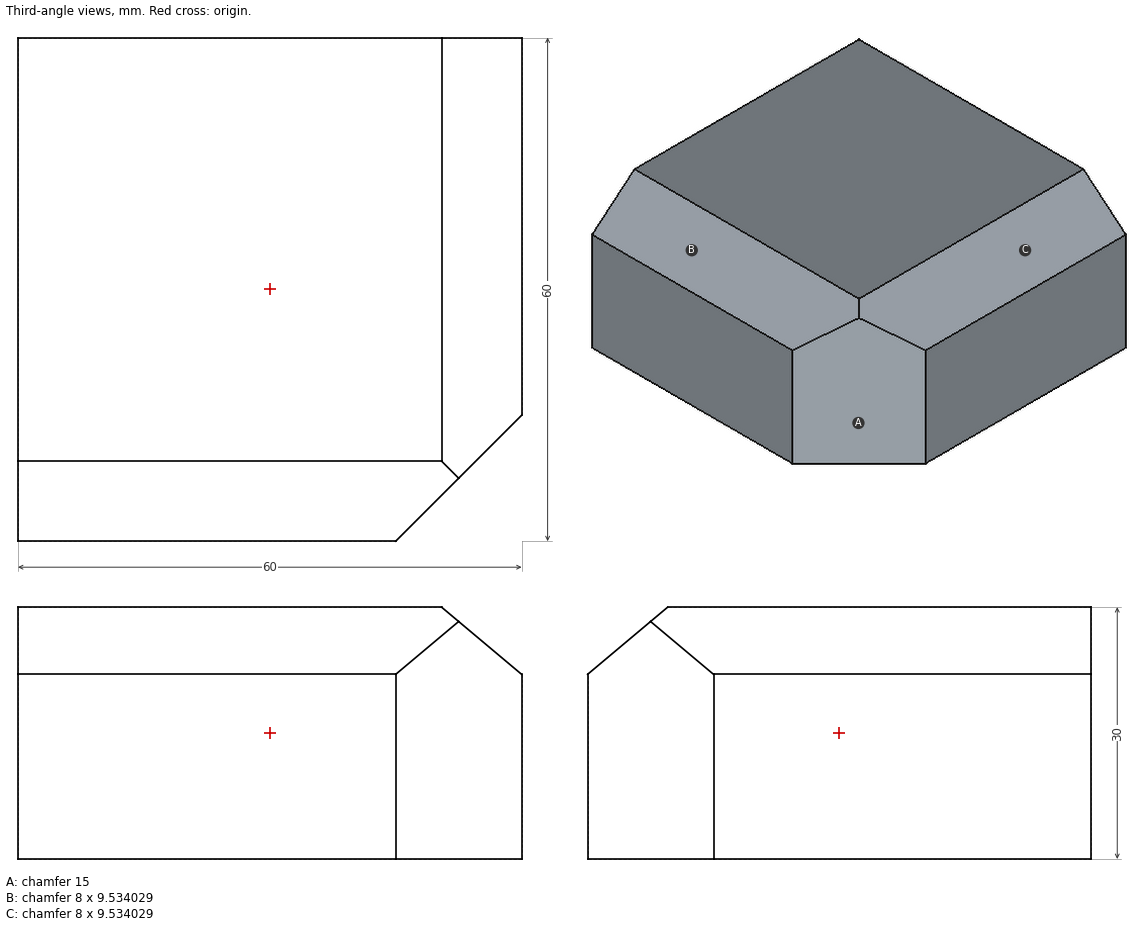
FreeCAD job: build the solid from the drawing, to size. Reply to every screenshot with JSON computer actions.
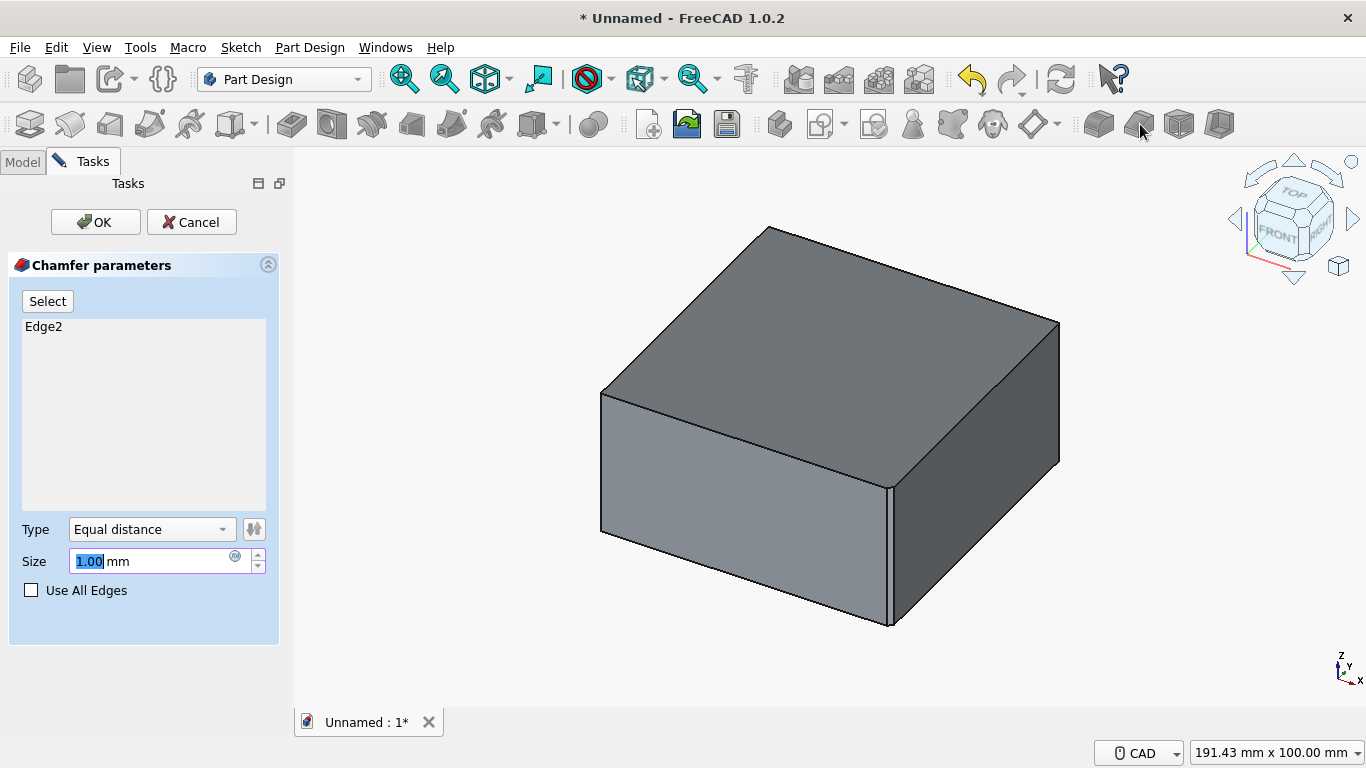
{"action": "type", "text": "15"}
{"action": "key", "text": "Tab"}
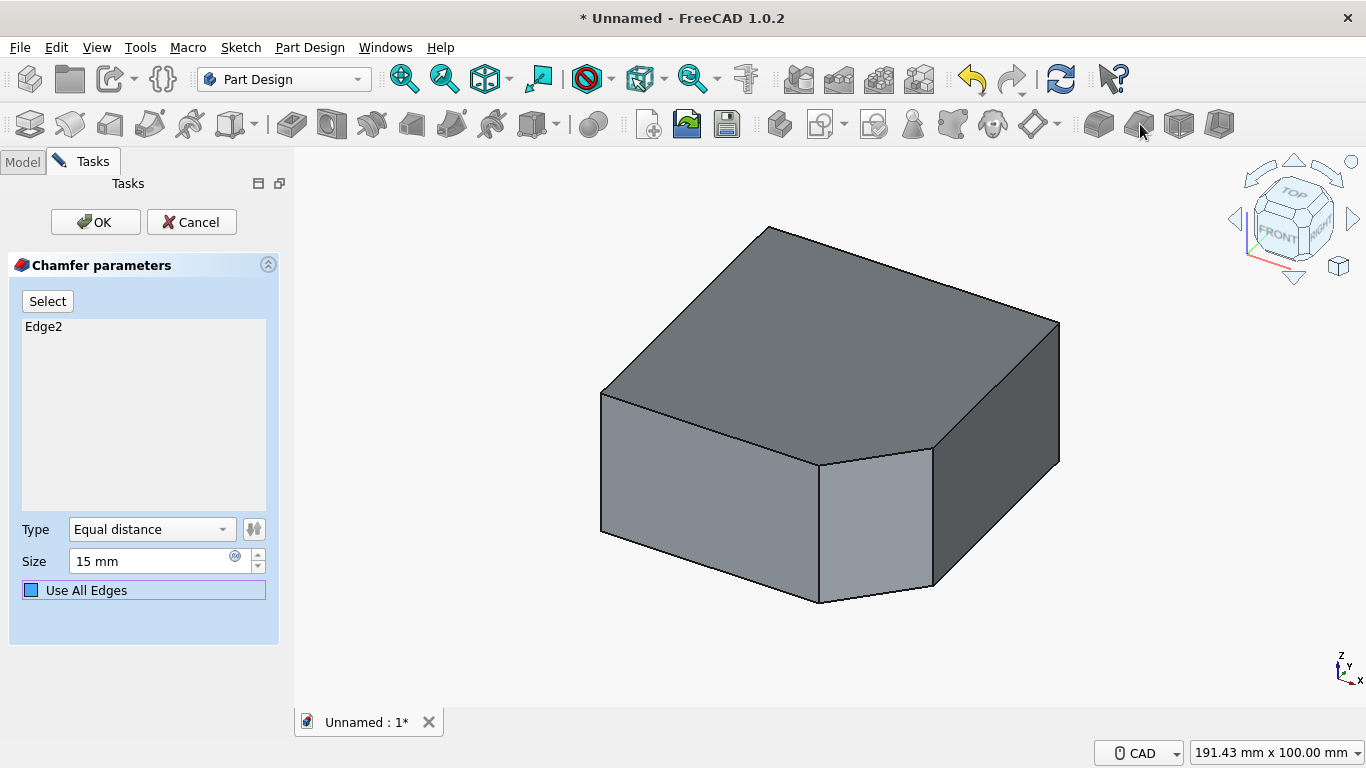
{"action": "left_click", "coordinate": [96, 222]}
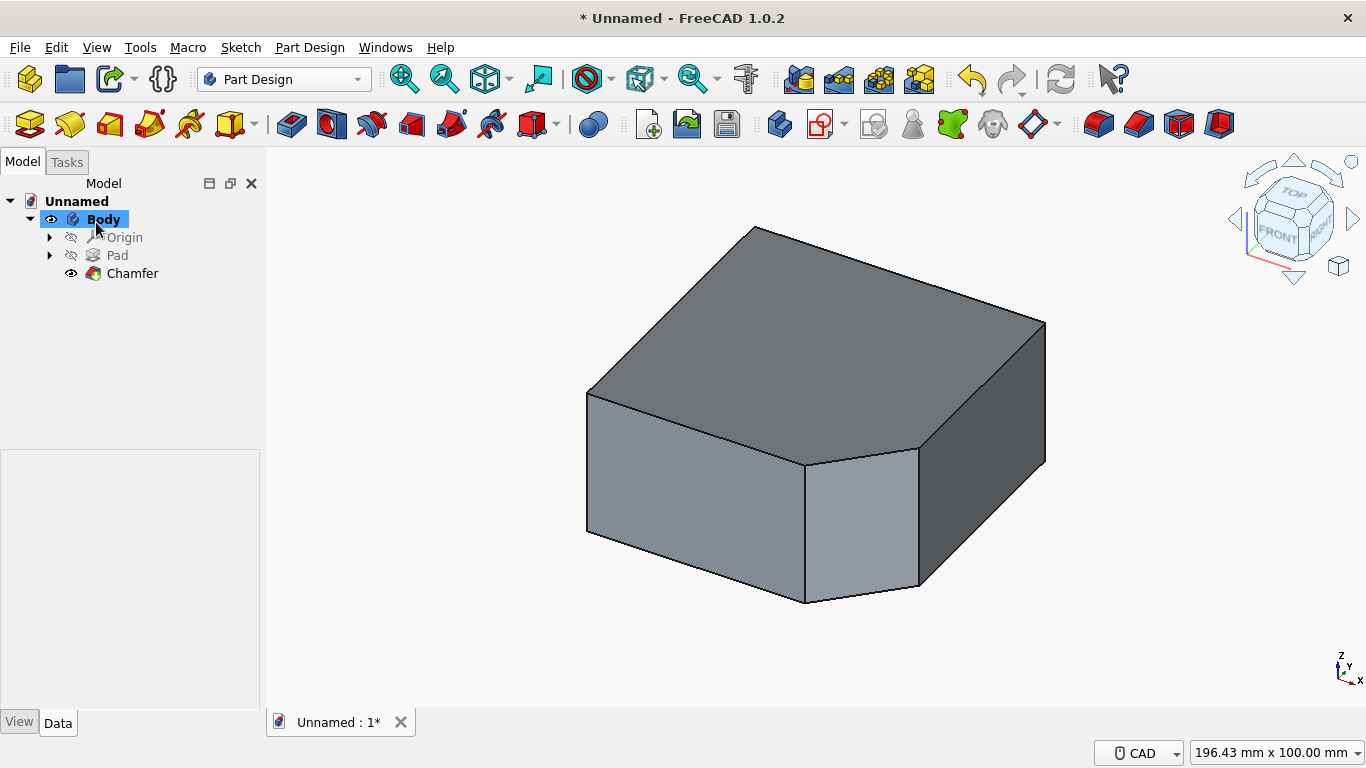
{"action": "left_click", "coordinate": [696, 429]}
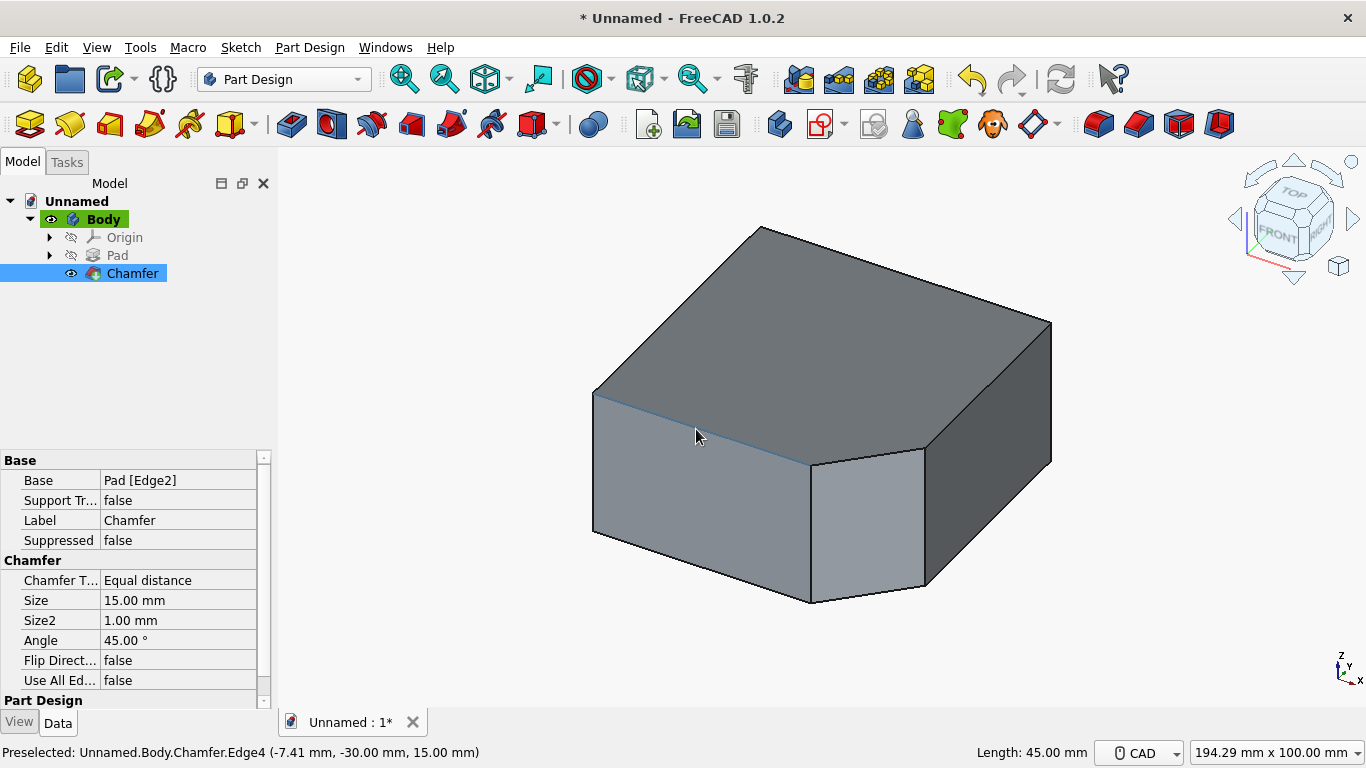
{"action": "left_click", "coordinate": [1140, 124]}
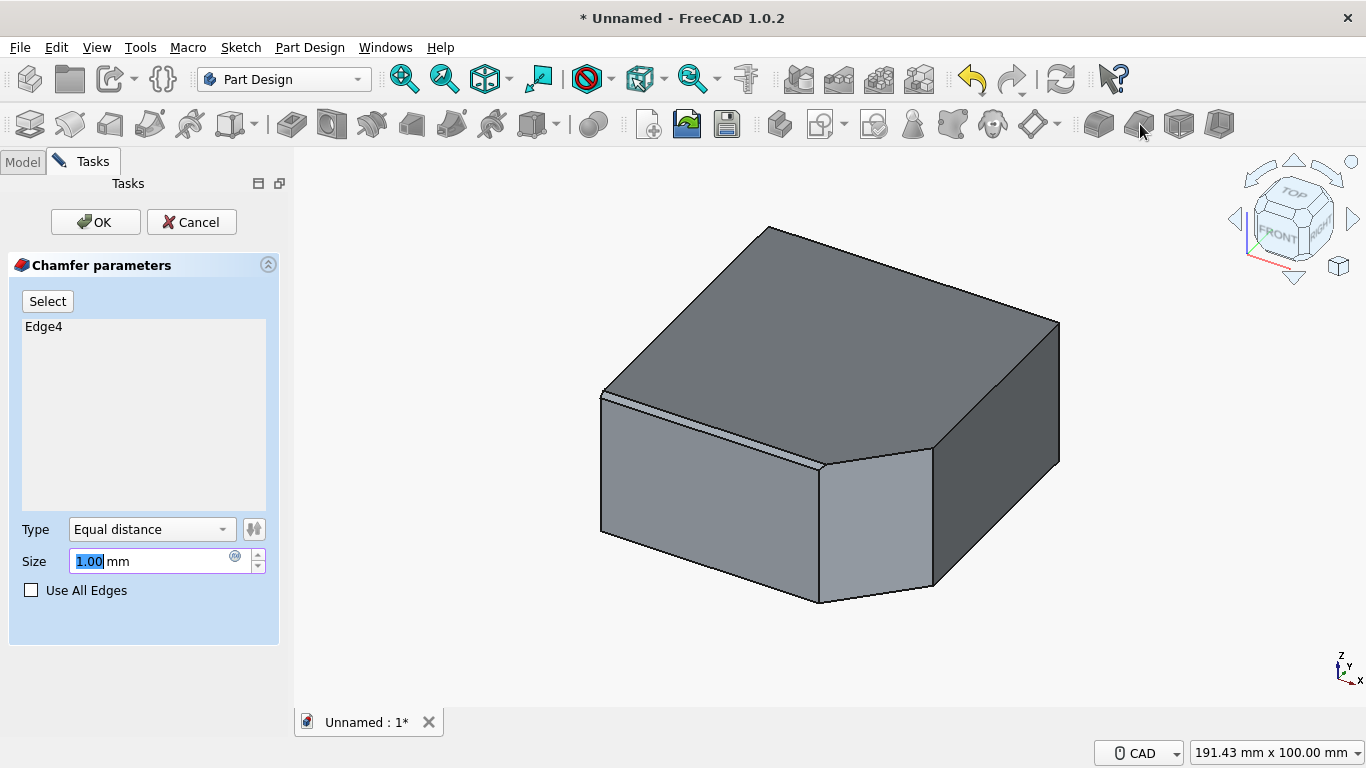
{"action": "type", "text": "8"}
{"action": "key", "text": "Tab"}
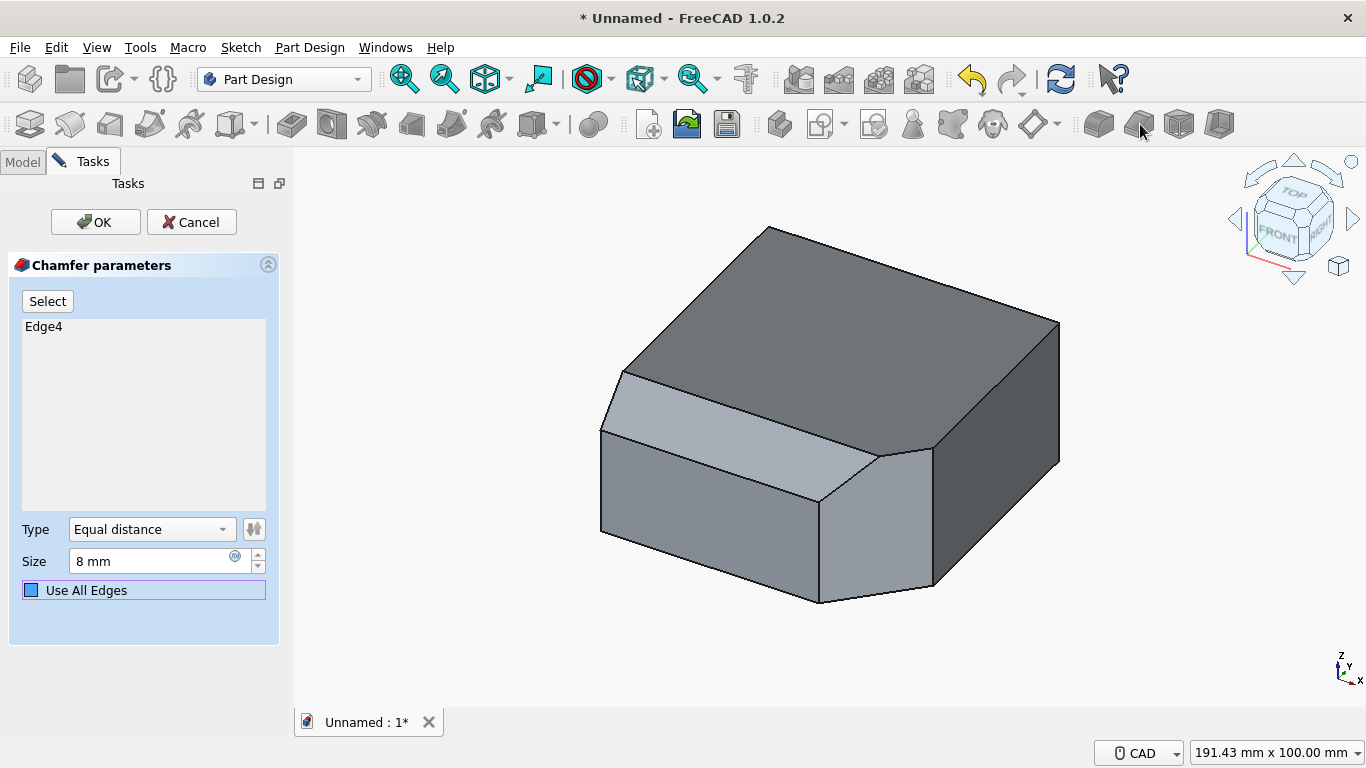
{"action": "left_click", "coordinate": [153, 530]}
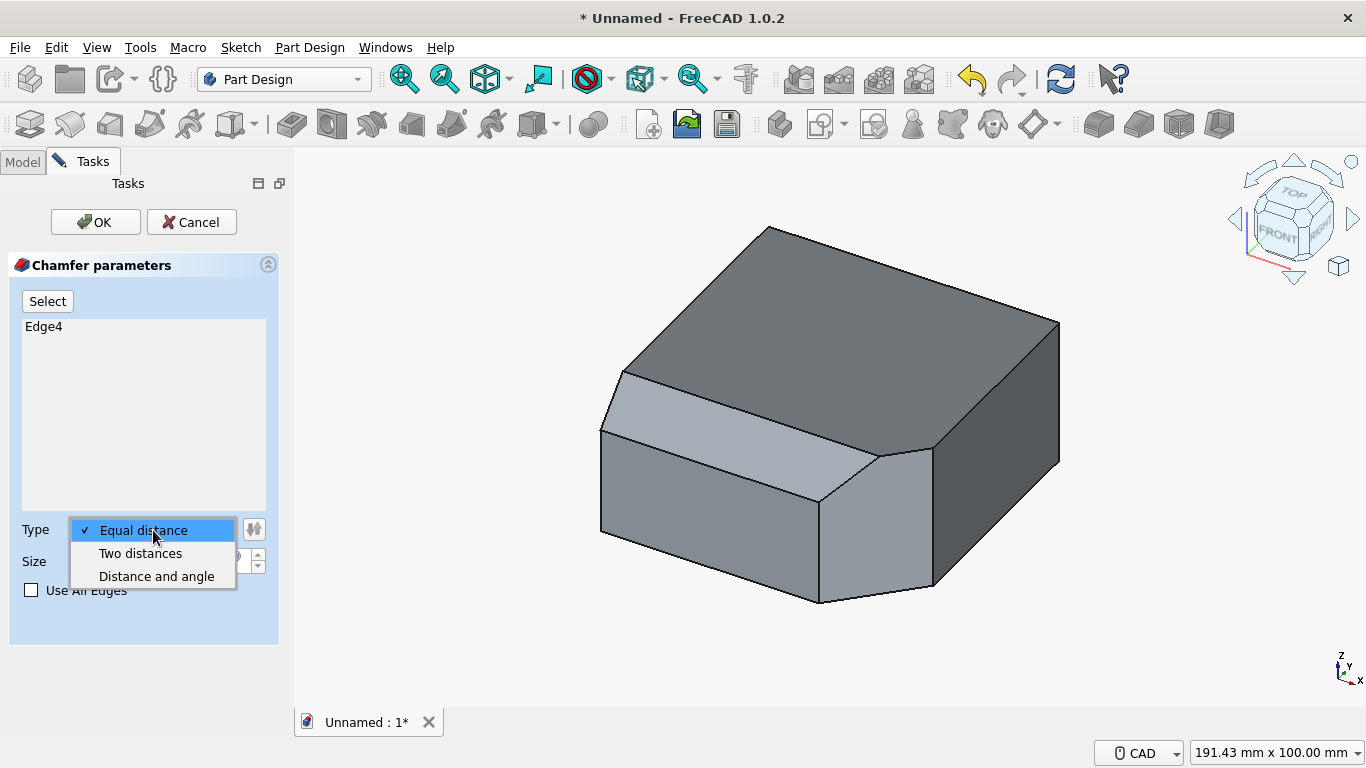
{"action": "left_click", "coordinate": [152, 554]}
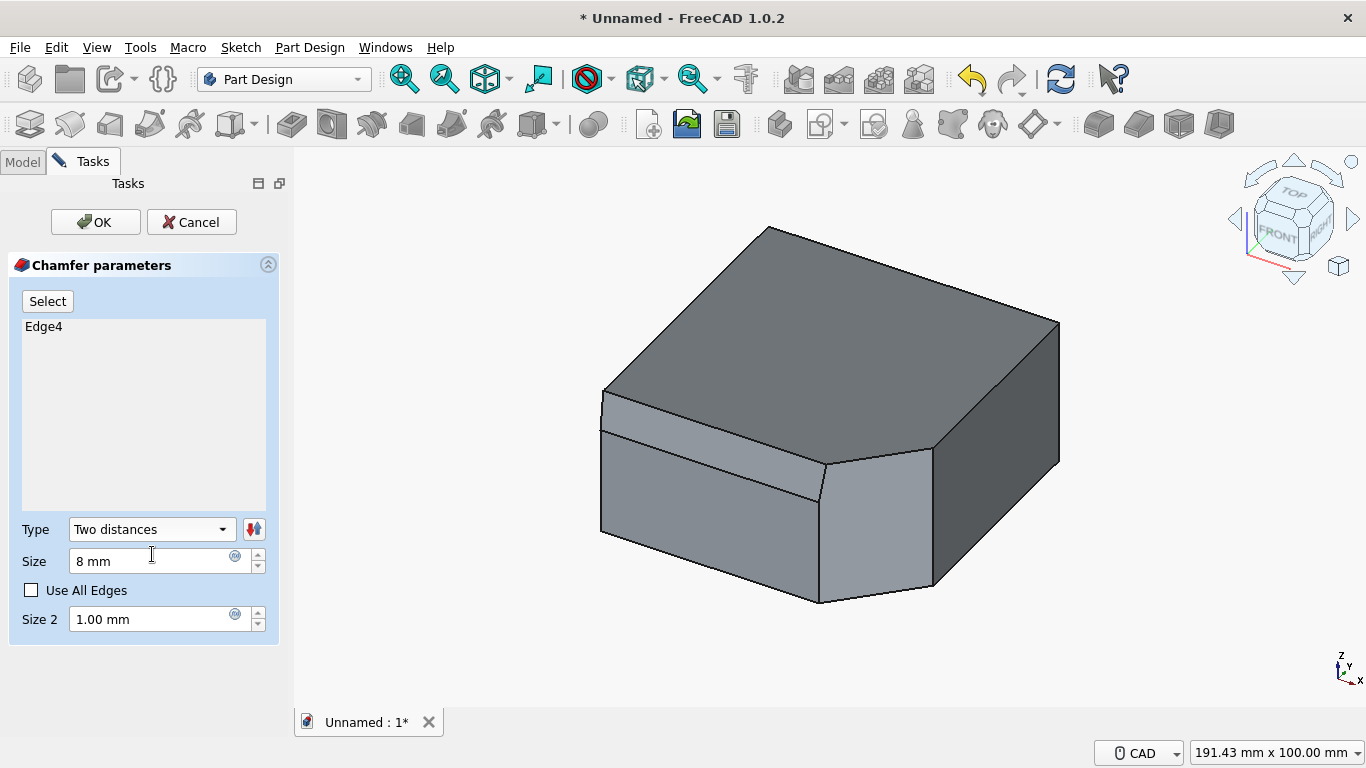
{"action": "triple_click", "coordinate": [160, 619]}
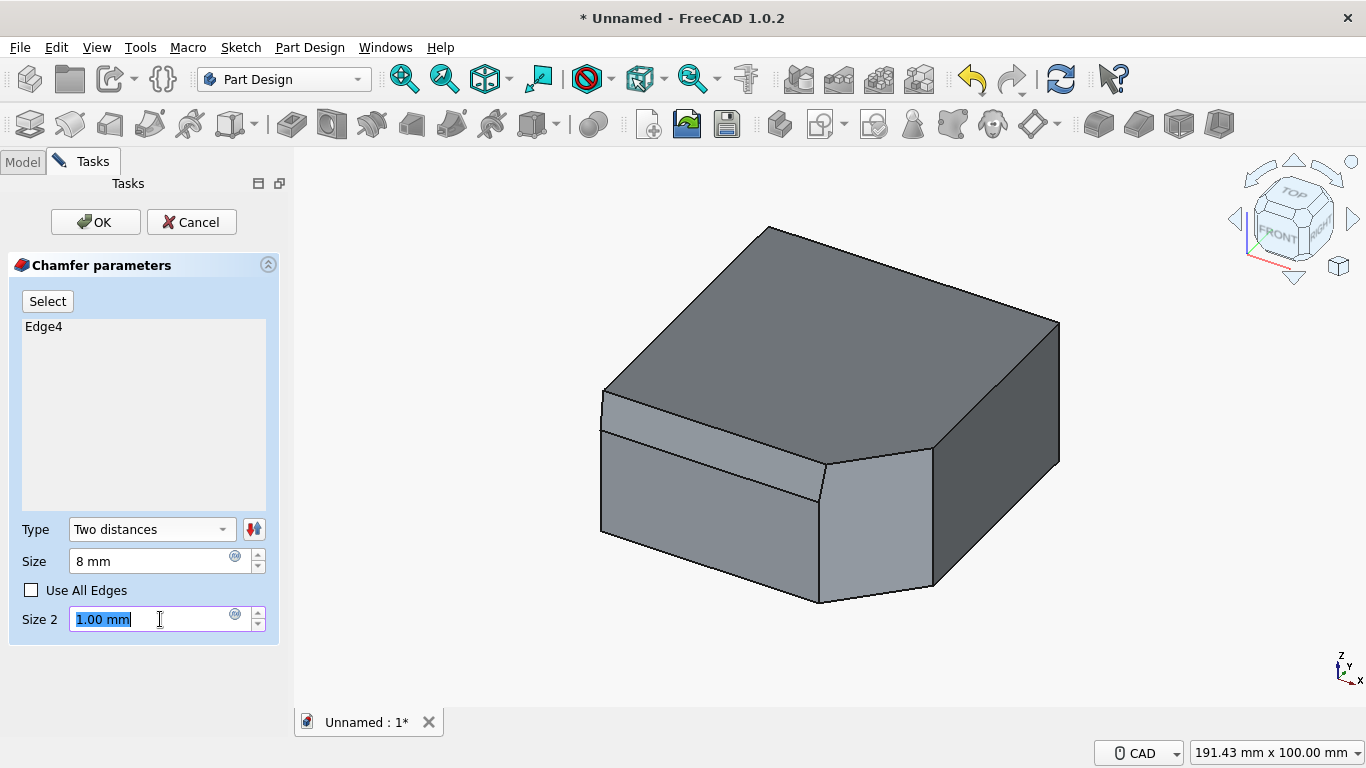
{"action": "type", "text": "9.534029"}
{"action": "key", "text": "Tab"}